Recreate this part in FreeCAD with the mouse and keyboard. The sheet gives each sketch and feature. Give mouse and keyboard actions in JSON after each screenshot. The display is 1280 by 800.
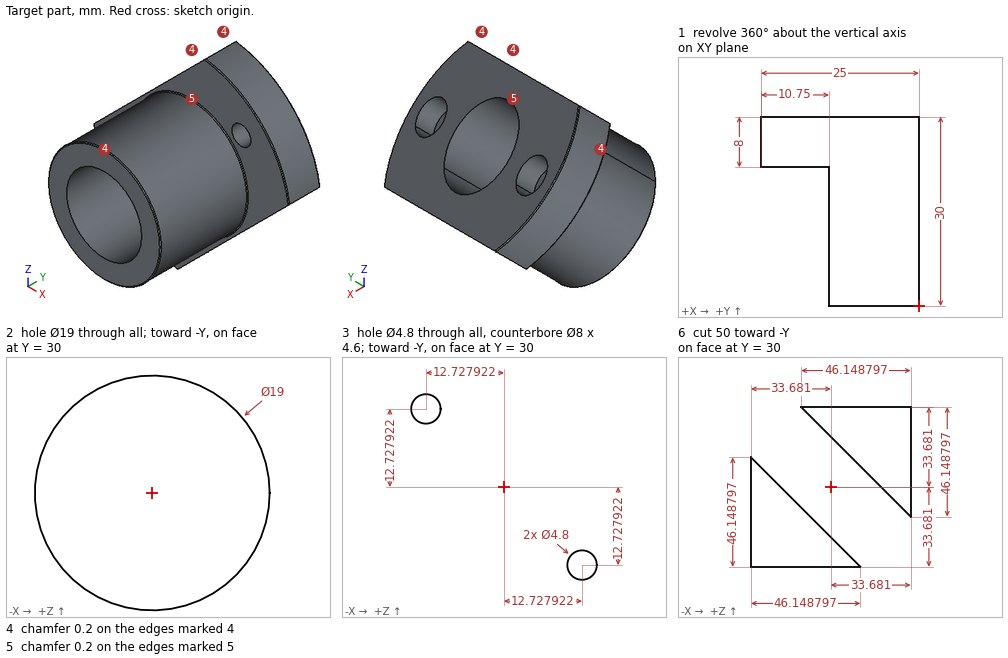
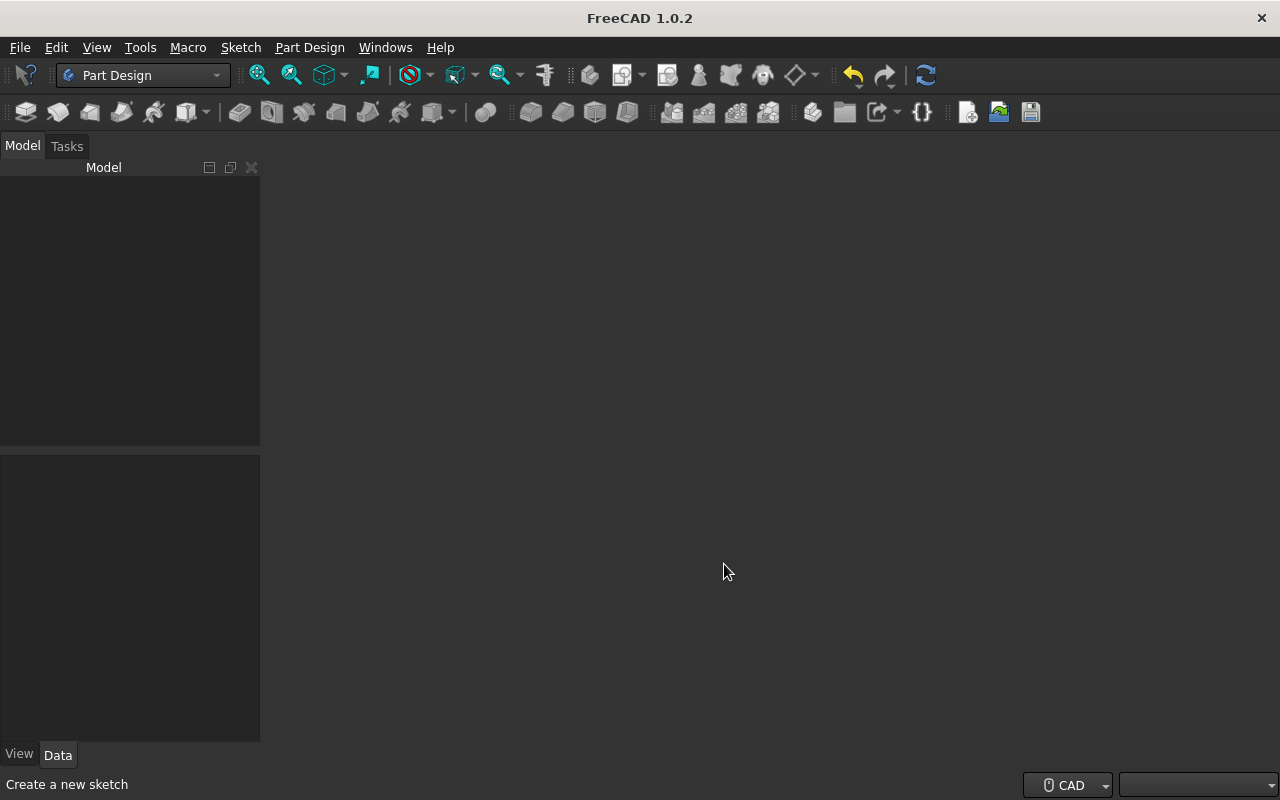
{"action": "left_click", "coordinate": [968, 112]}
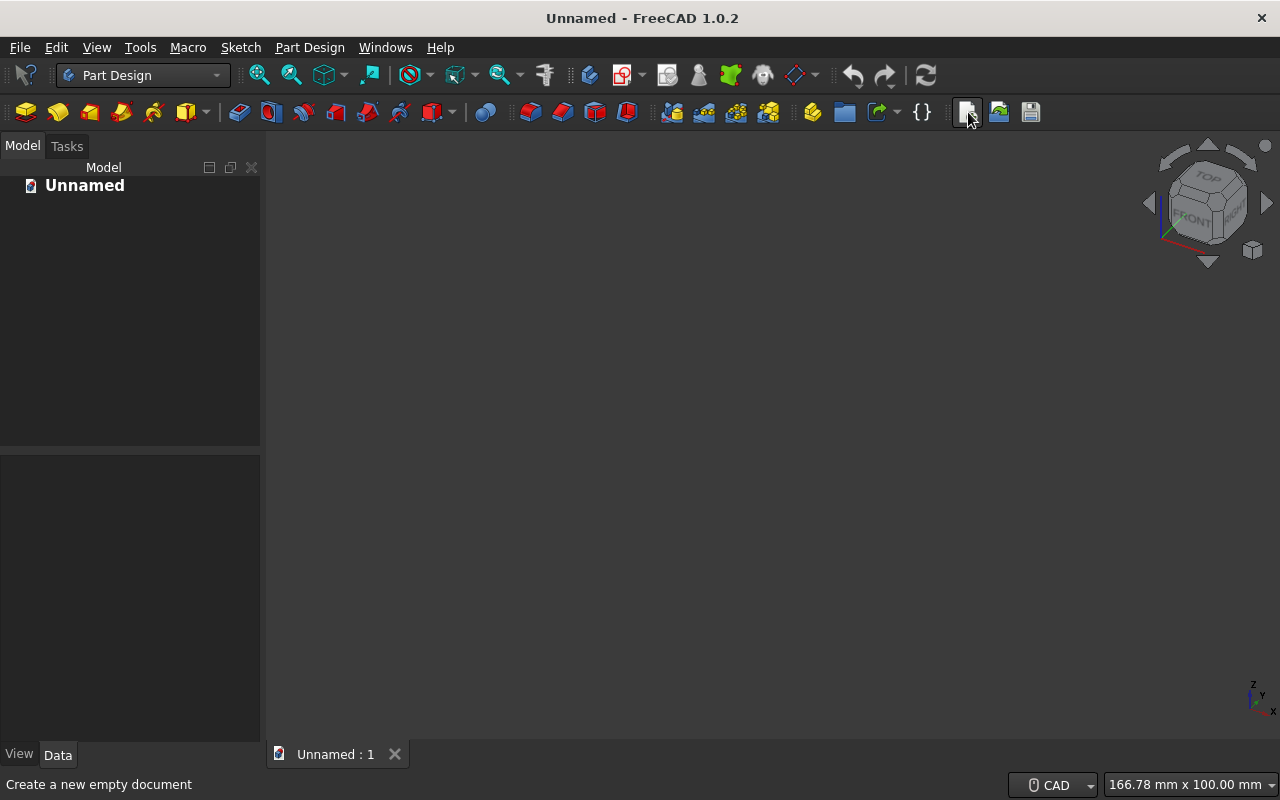
{"action": "left_click", "coordinate": [622, 76]}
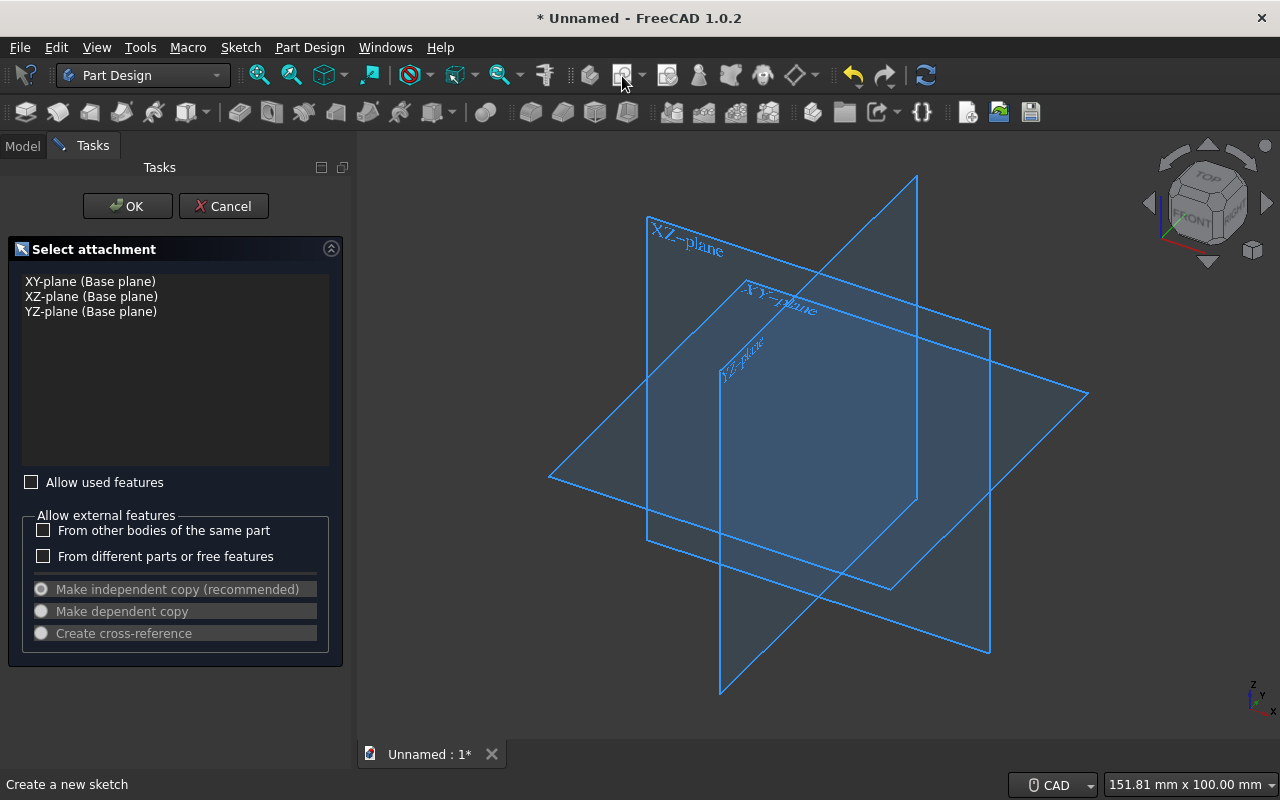
{"action": "left_click", "coordinate": [82, 282]}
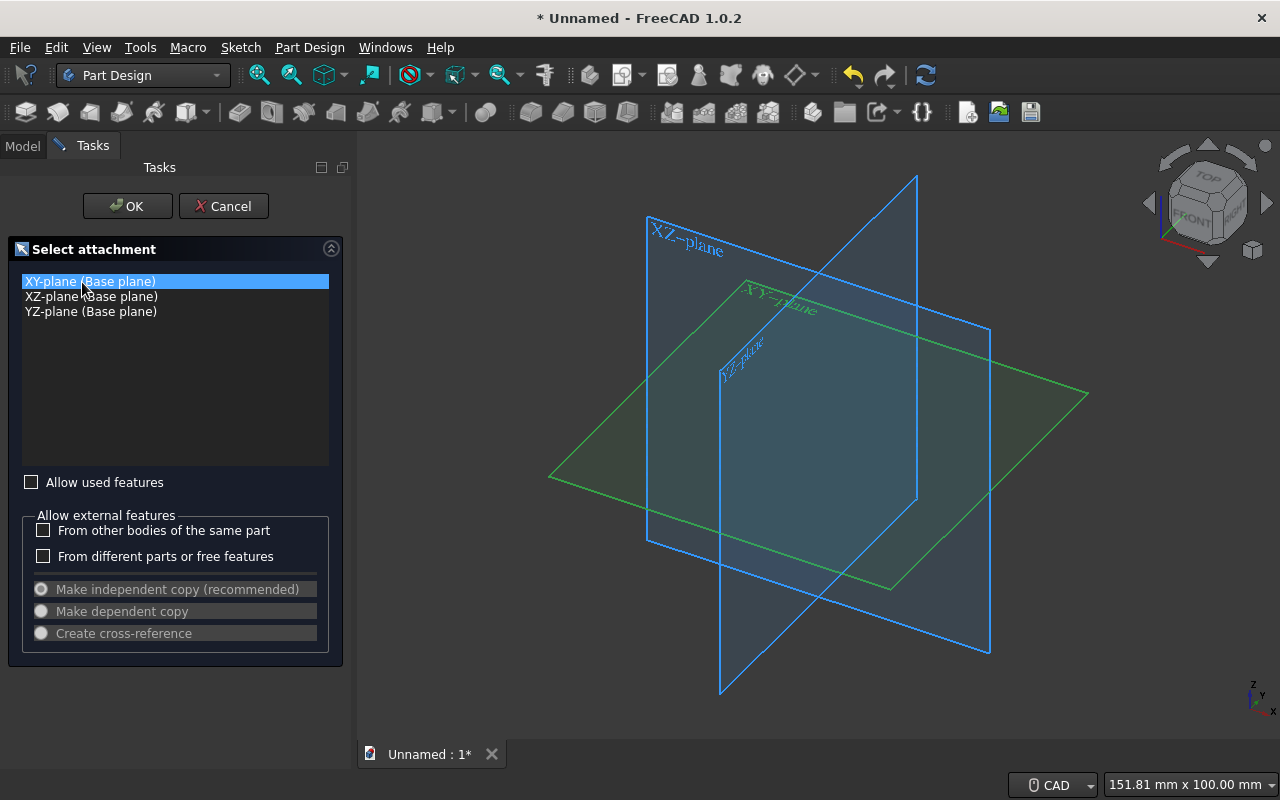
{"action": "left_click", "coordinate": [128, 206]}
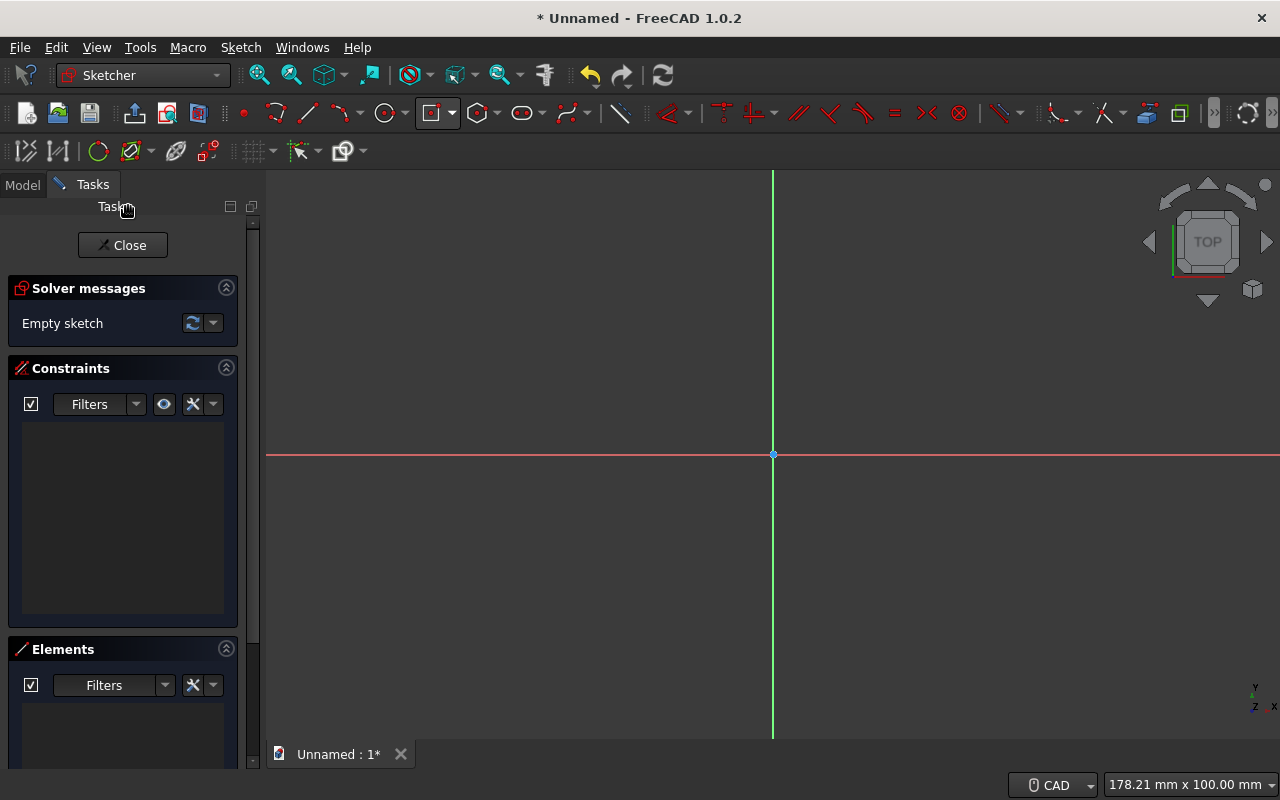
{"action": "scroll", "coordinate": [700, 300], "scroll_direction": "up", "scroll_amount": 4}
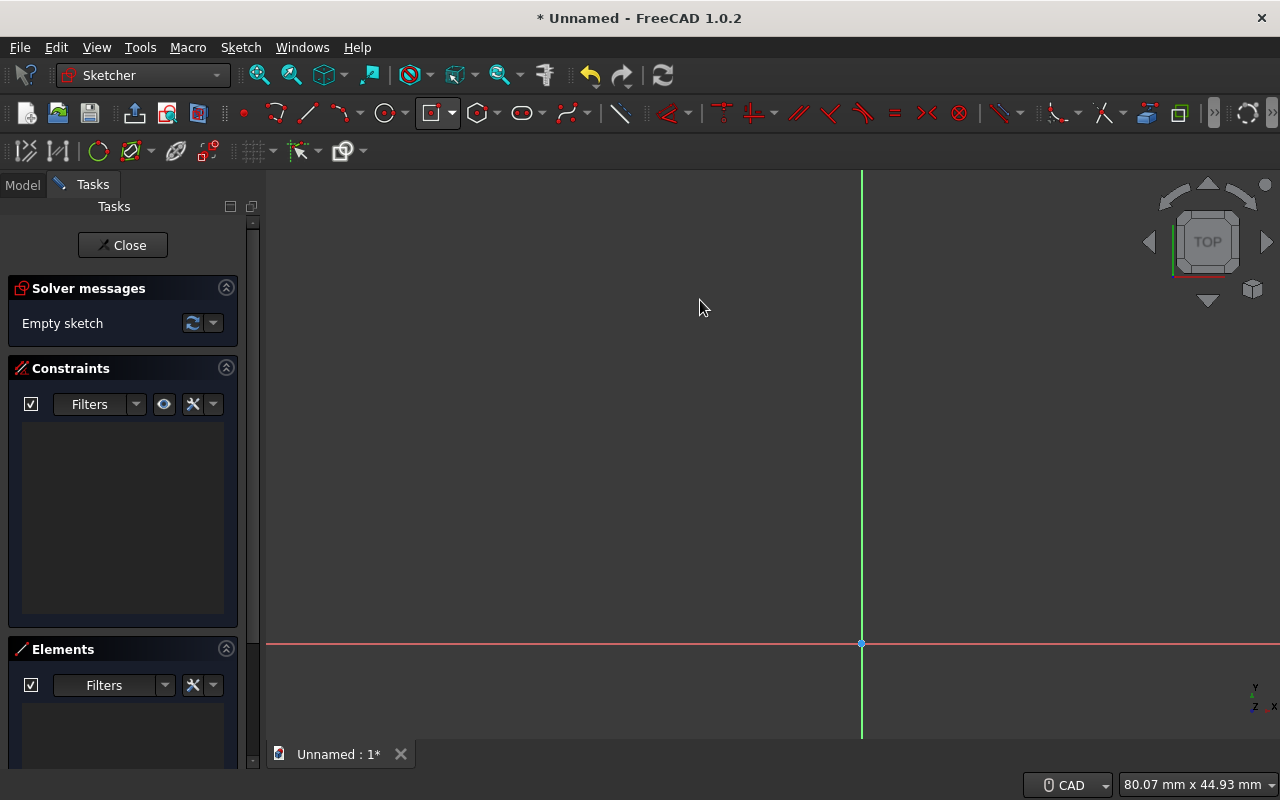
{"action": "left_click", "coordinate": [276, 114]}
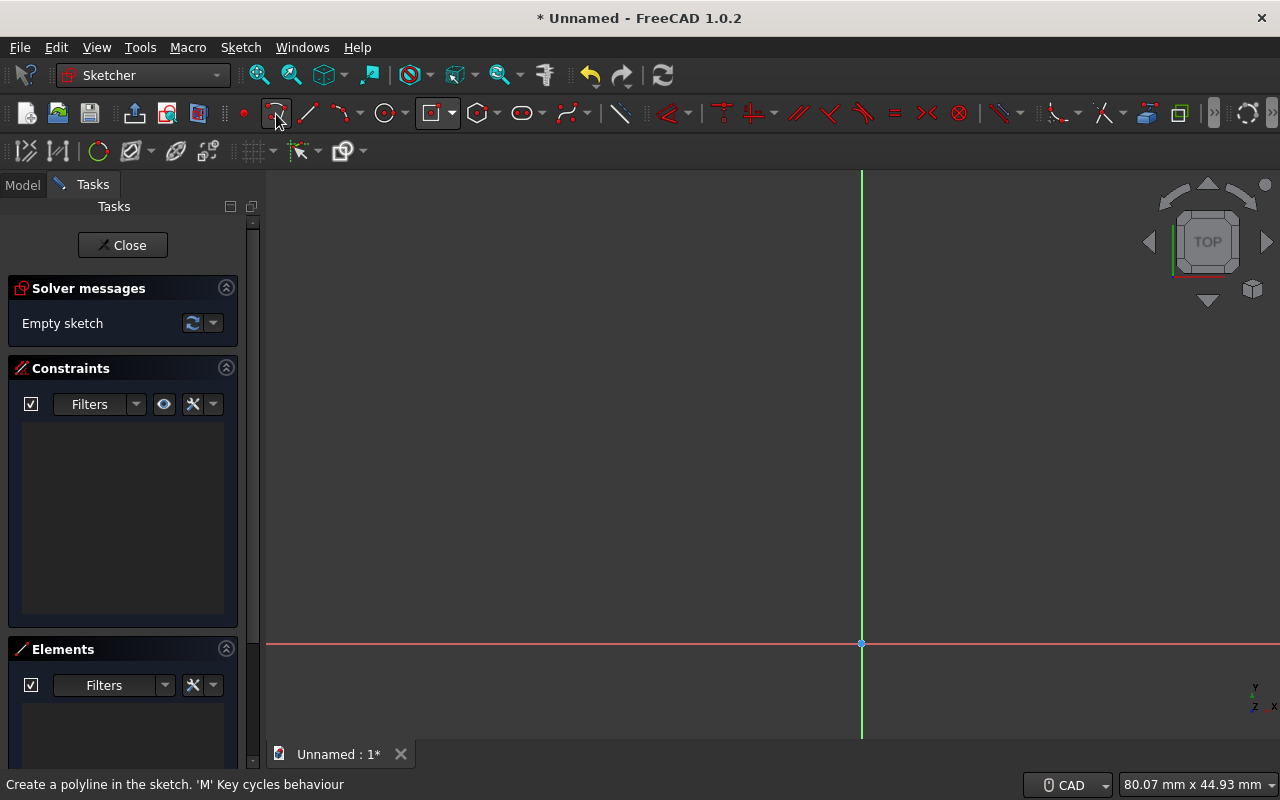
{"action": "left_click", "coordinate": [862, 644]}
{"action": "left_click", "coordinate": [853, 264]}
{"action": "left_click", "coordinate": [545, 264]}
{"action": "left_click", "coordinate": [545, 365]}
{"action": "left_click", "coordinate": [681, 365]}
{"action": "left_click", "coordinate": [681, 635]}
{"action": "left_click", "coordinate": [862, 644]}
{"action": "key", "text": "Escape"}
{"action": "key", "text": "Escape"}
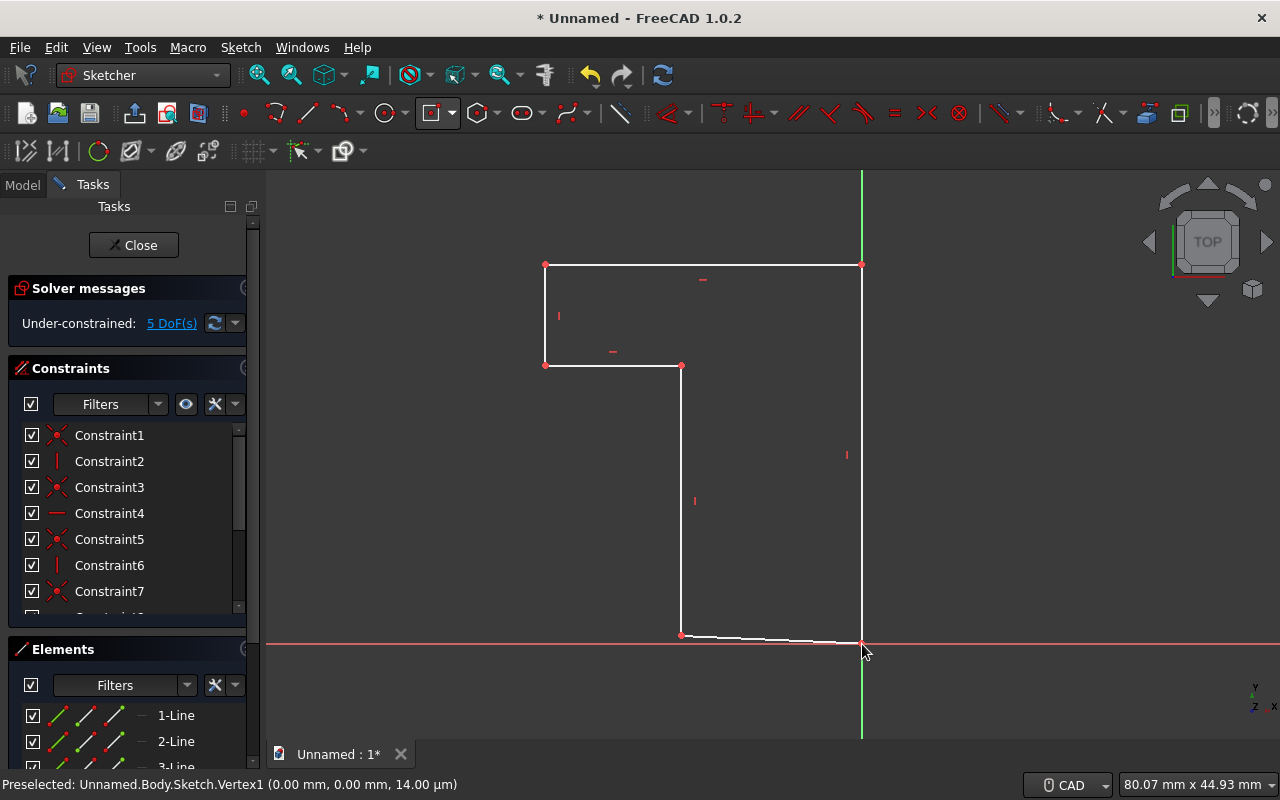
{"action": "left_click", "coordinate": [808, 641]}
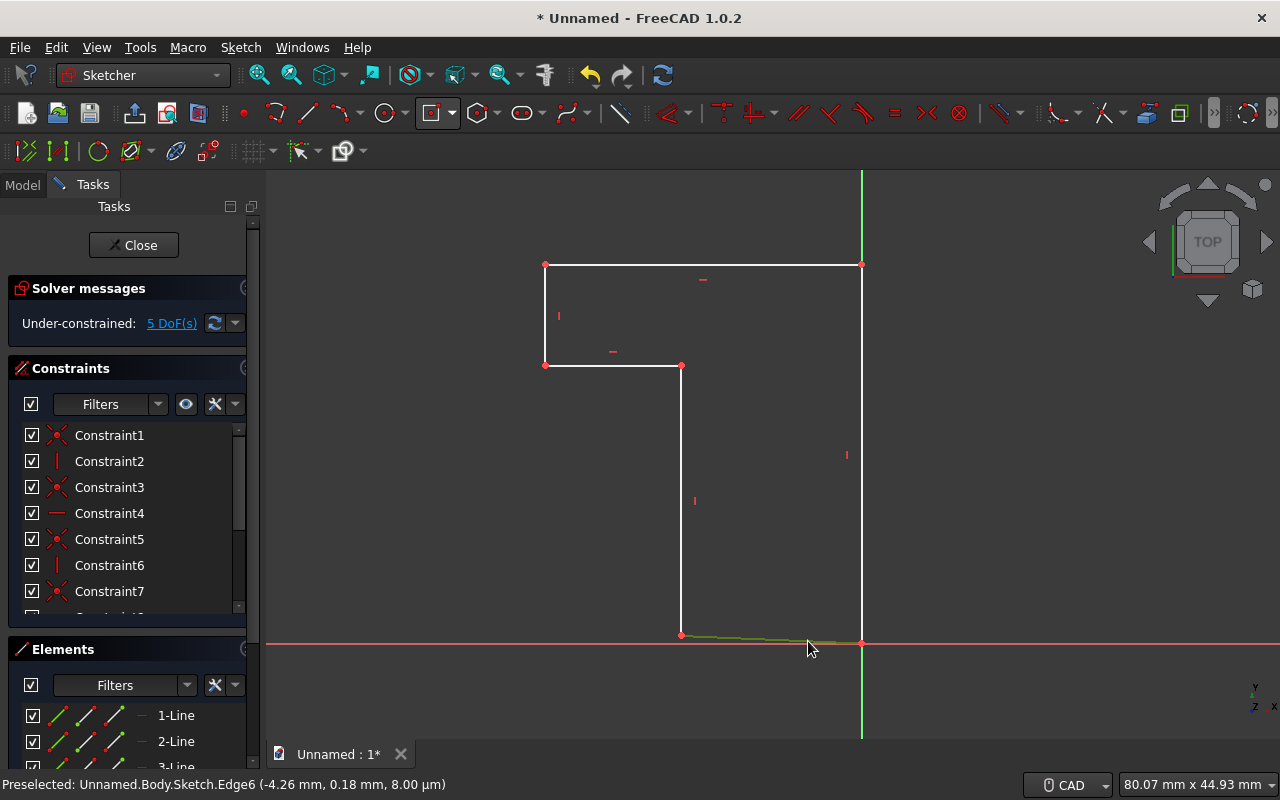
{"action": "left_click", "coordinate": [776, 114]}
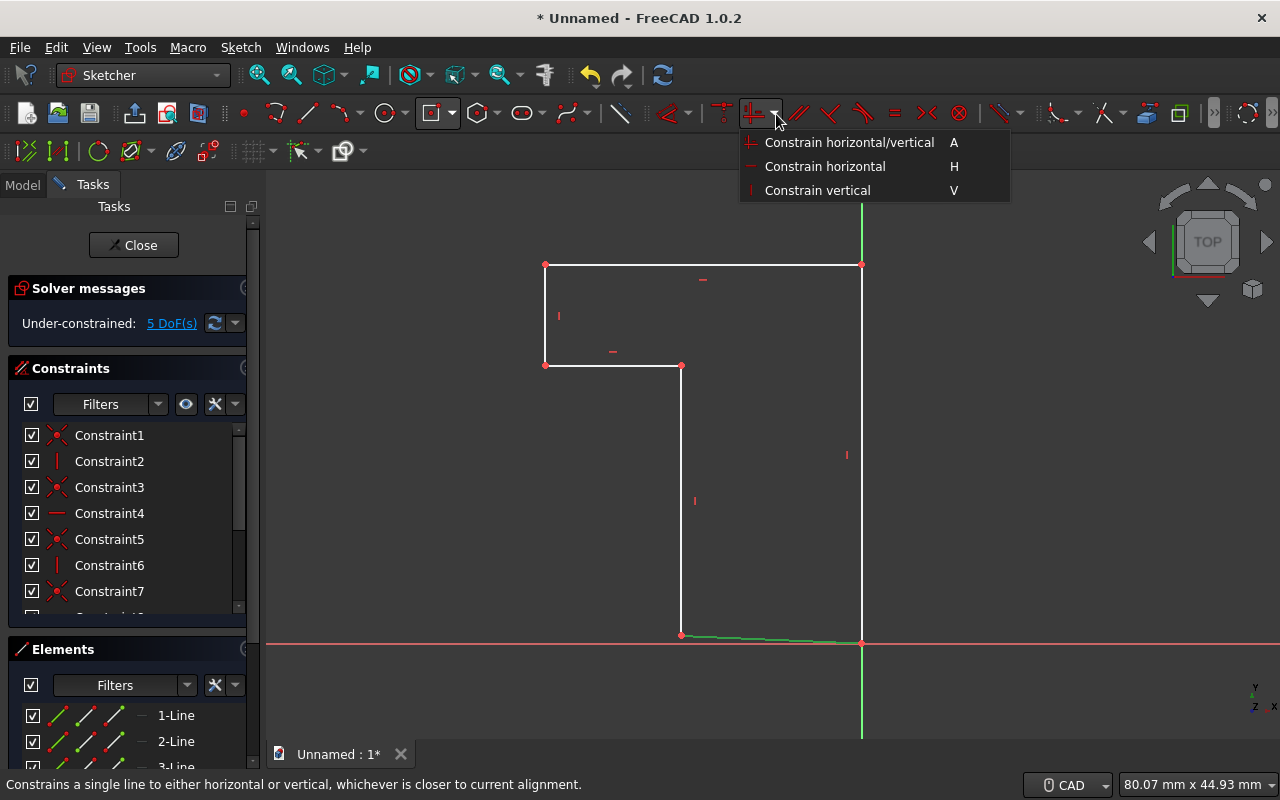
{"action": "left_click", "coordinate": [875, 166]}